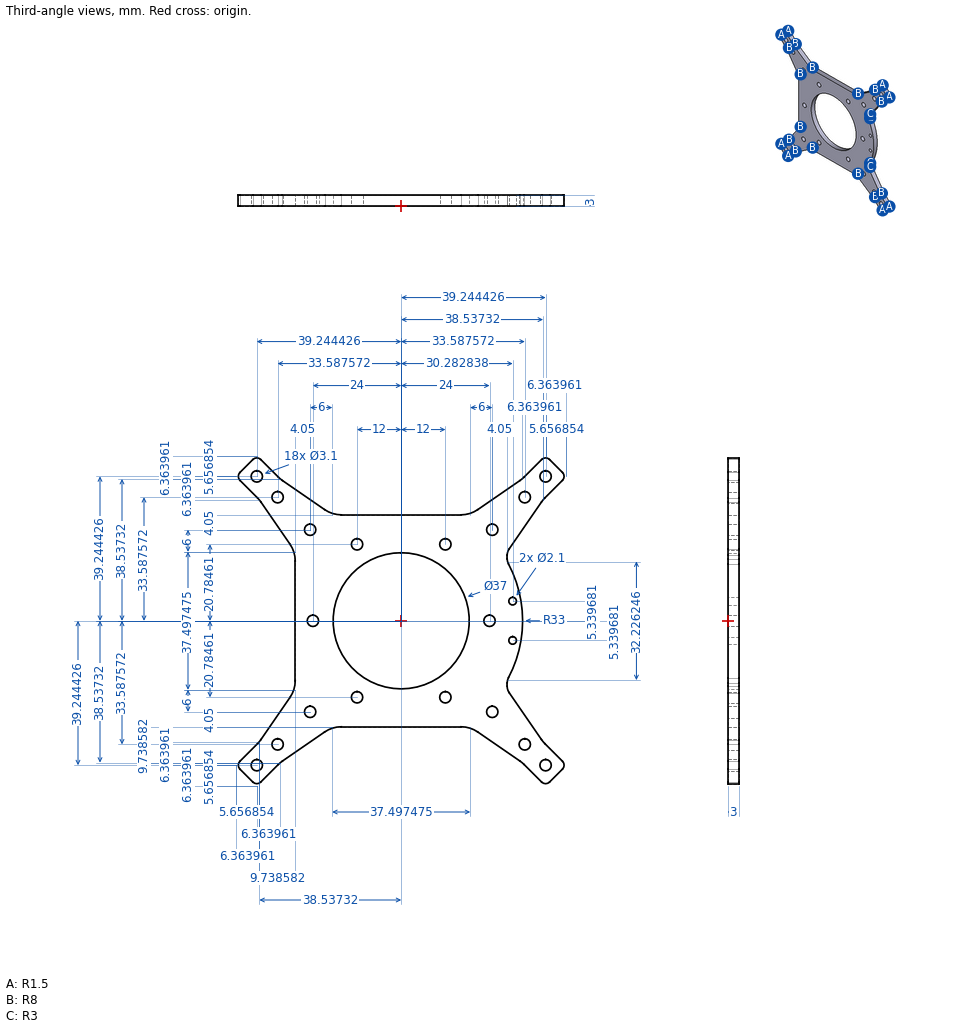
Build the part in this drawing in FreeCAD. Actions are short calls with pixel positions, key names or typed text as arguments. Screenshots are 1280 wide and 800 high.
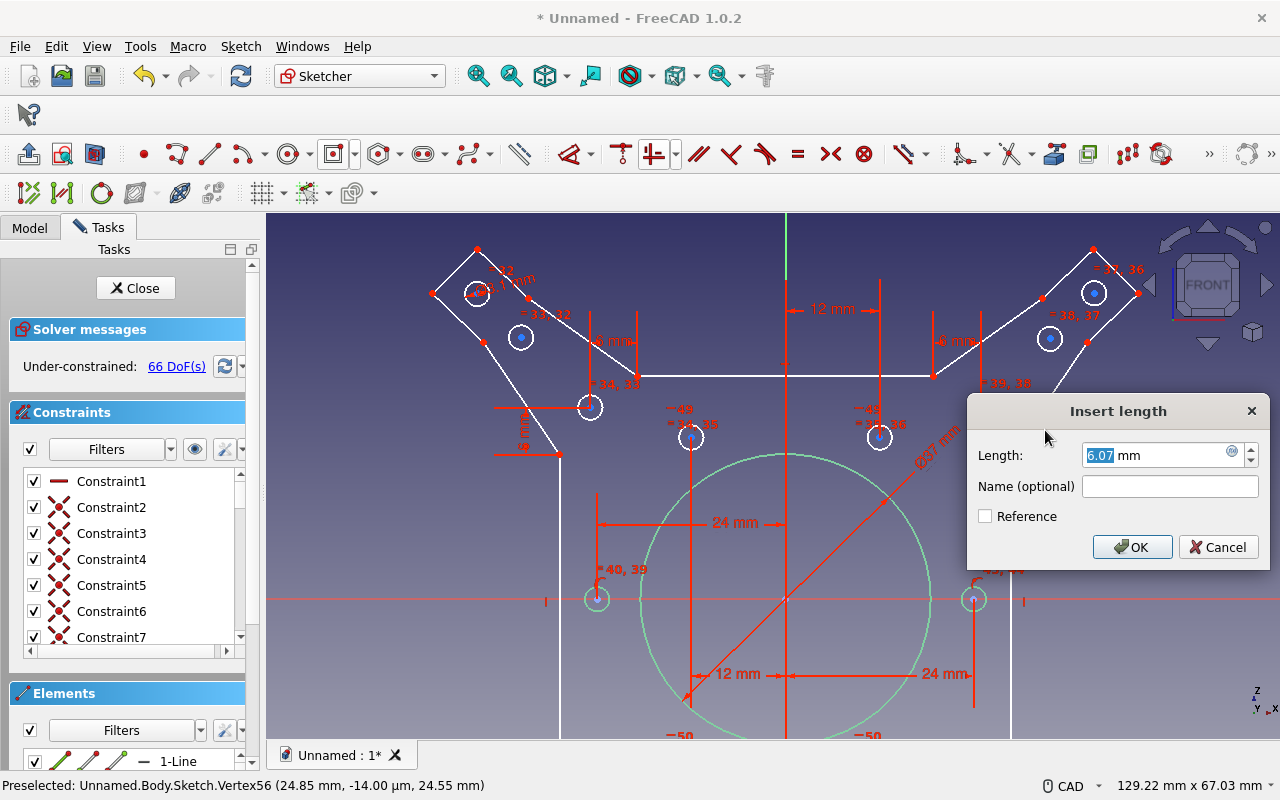
text(6)
key(Return)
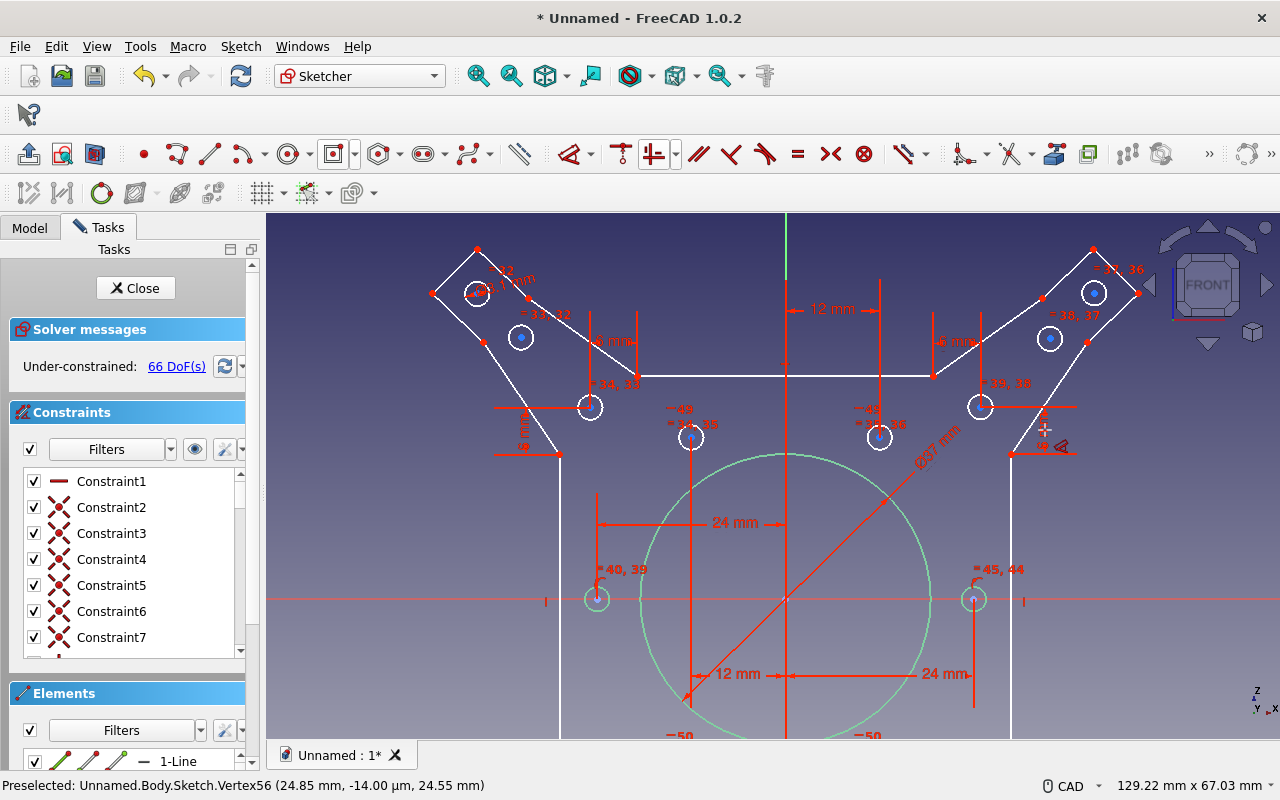
scroll(638, 375, down, 4)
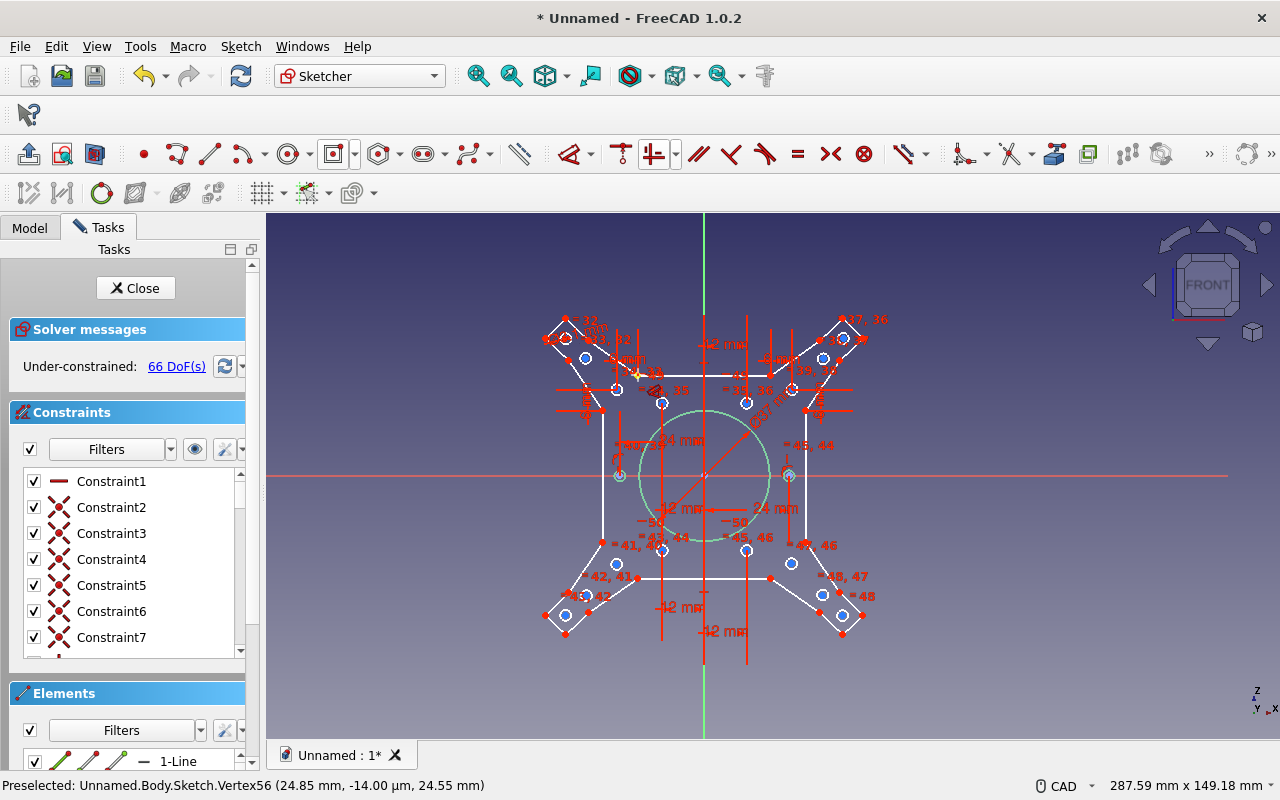
scroll(638, 579, up, 4)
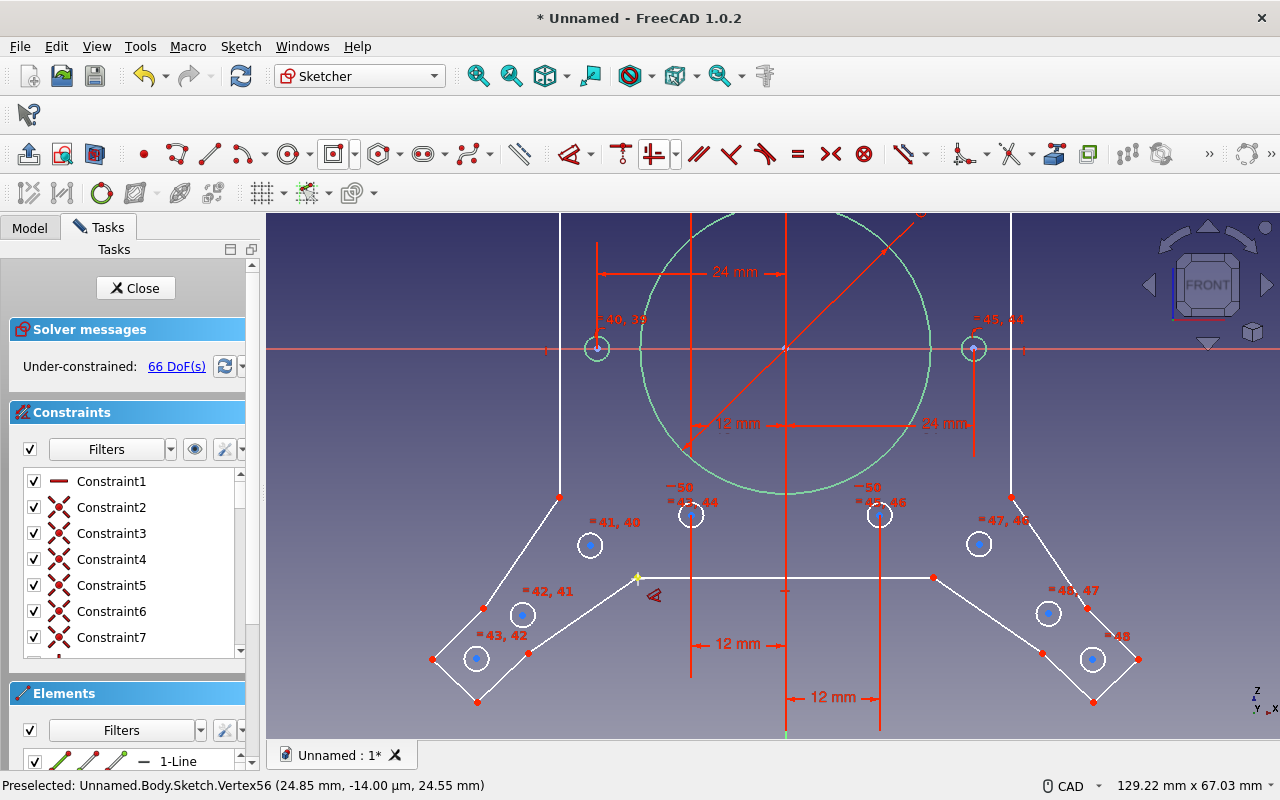
click(637, 578)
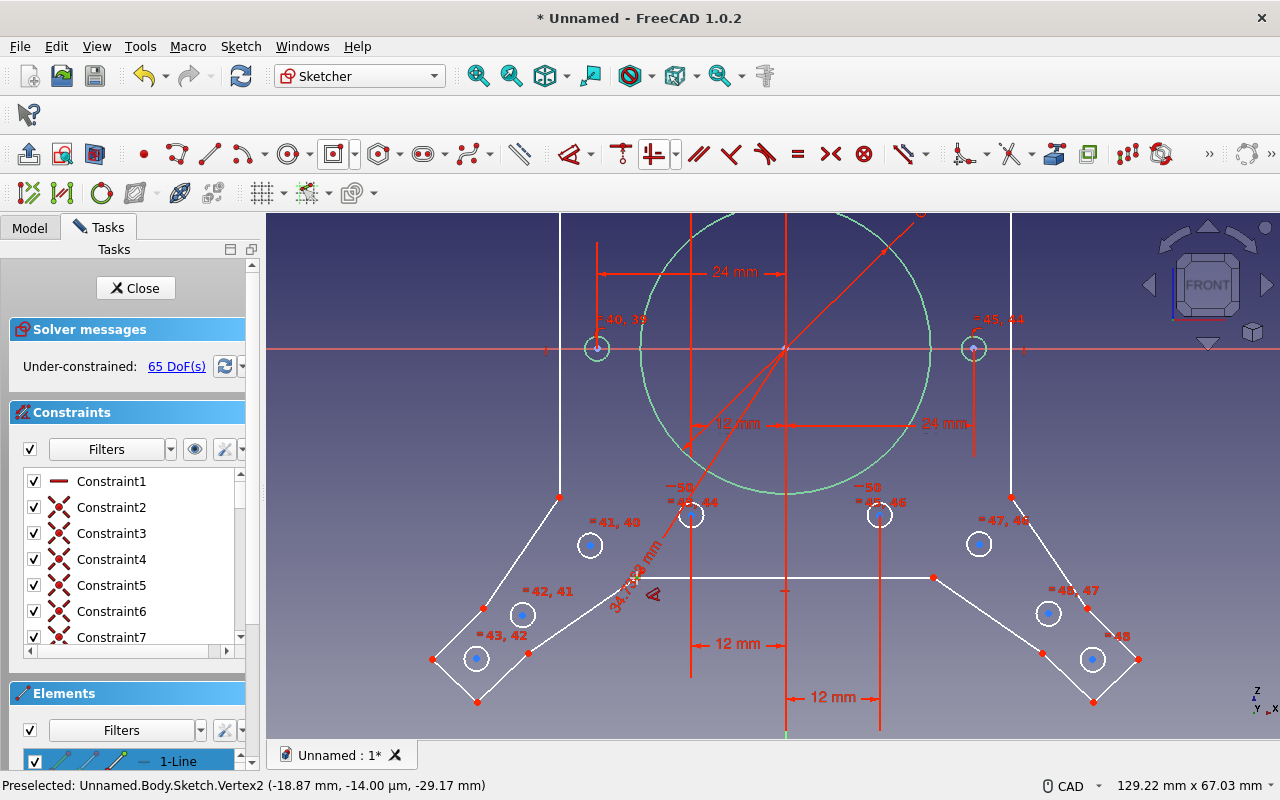
click(590, 546)
click(614, 612)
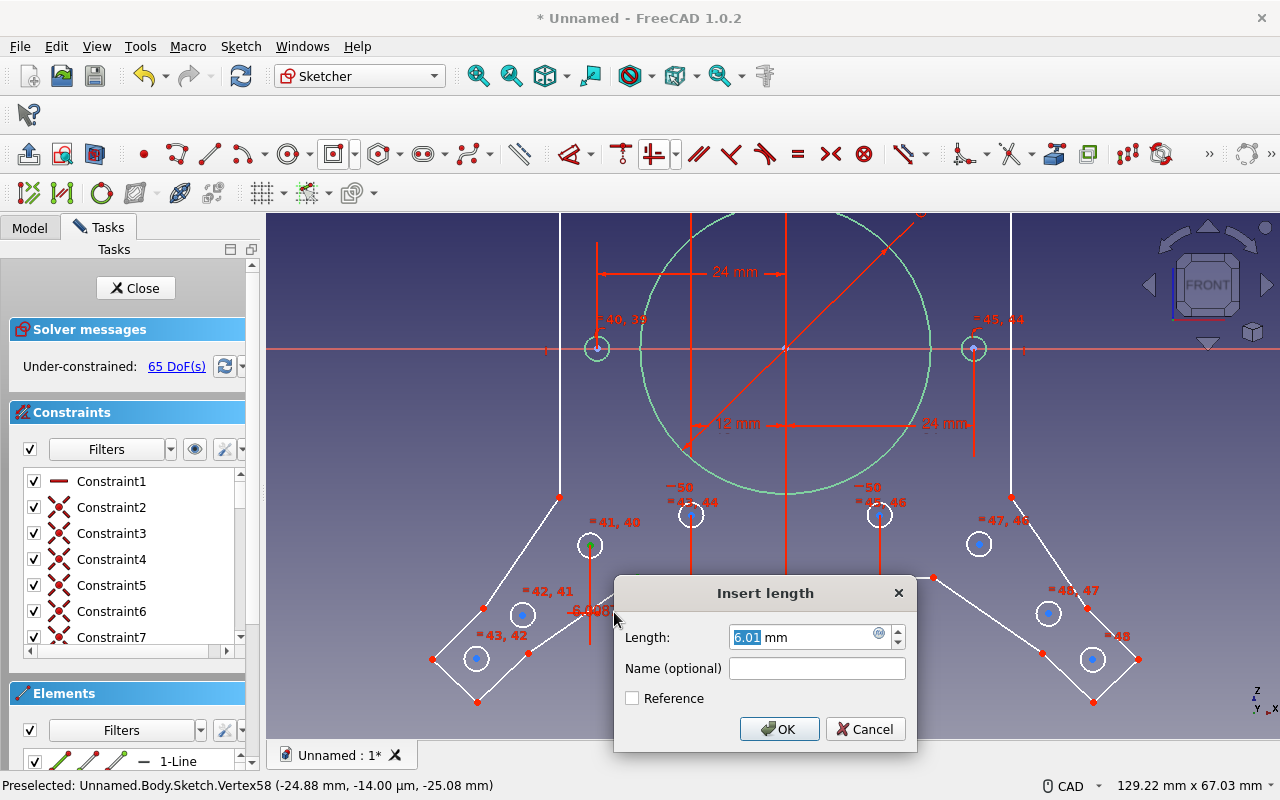
text(6)
key(Return)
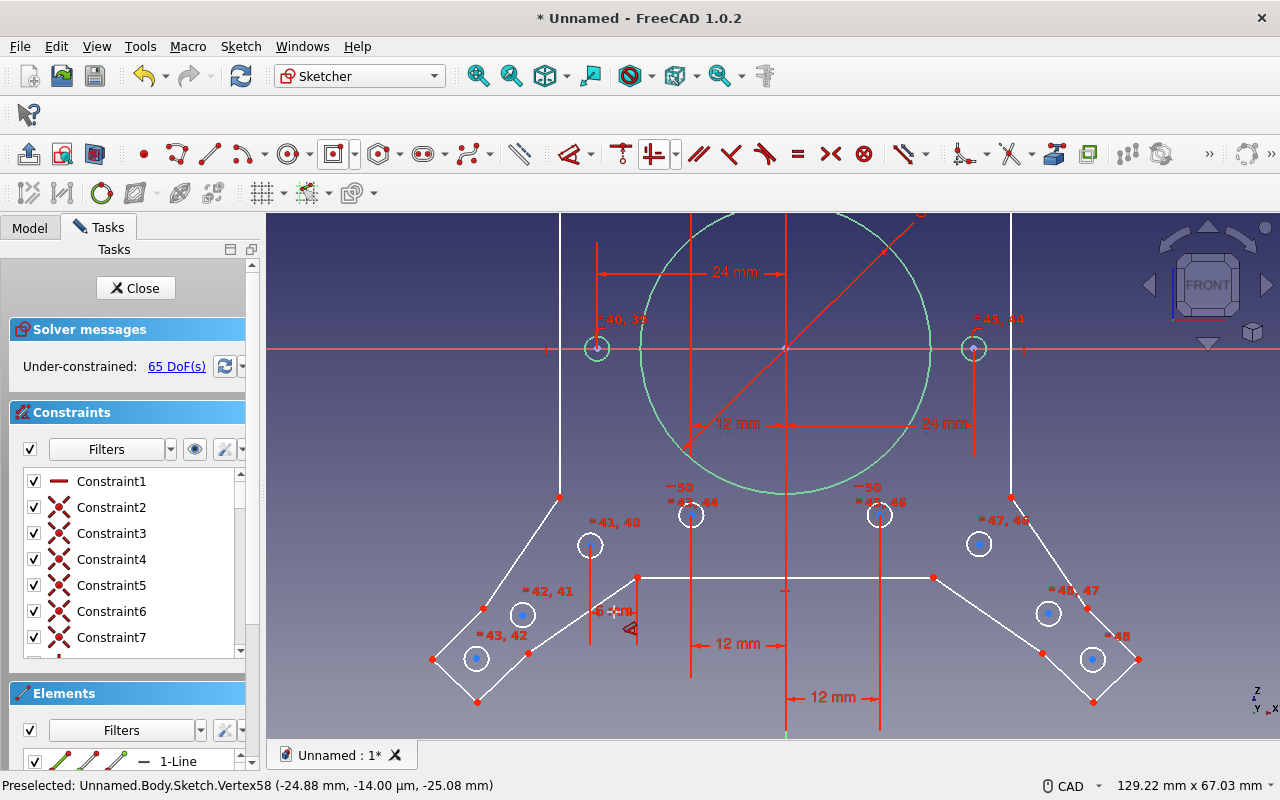
click(560, 498)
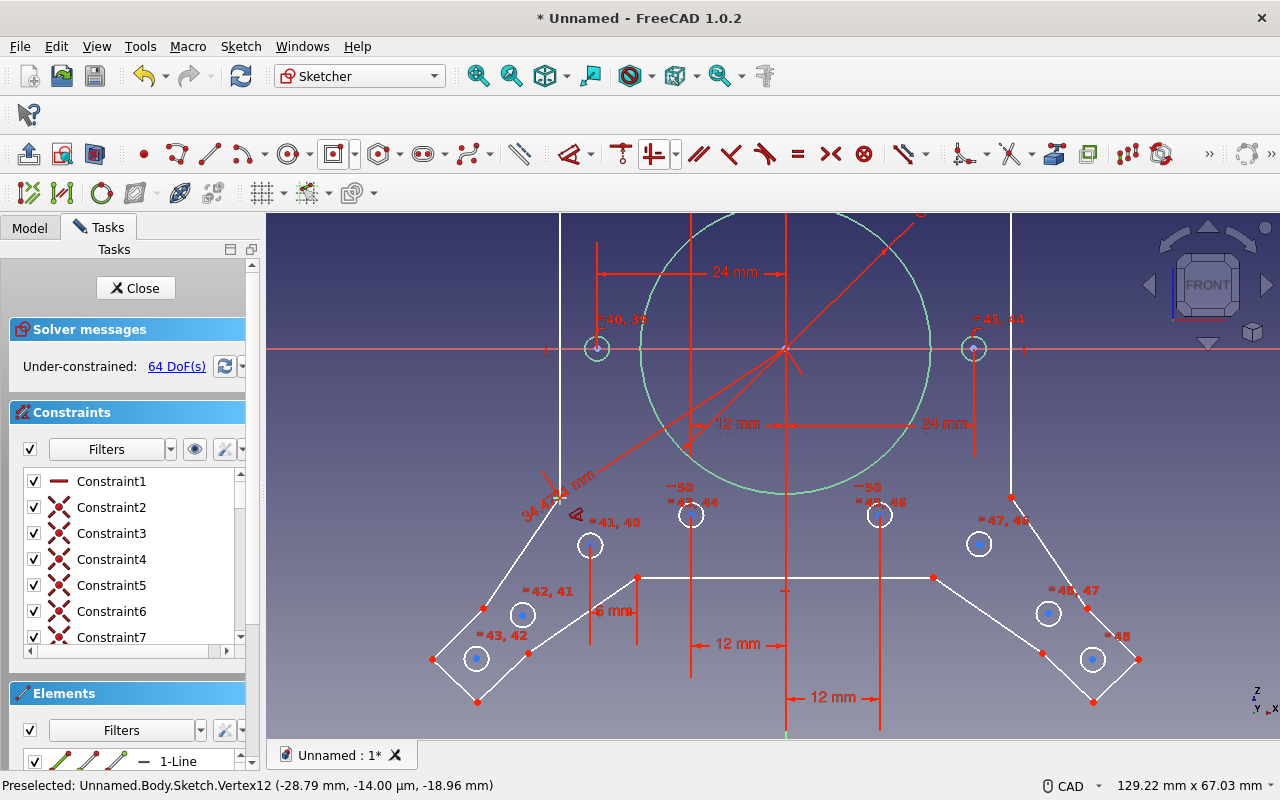
click(590, 546)
click(526, 522)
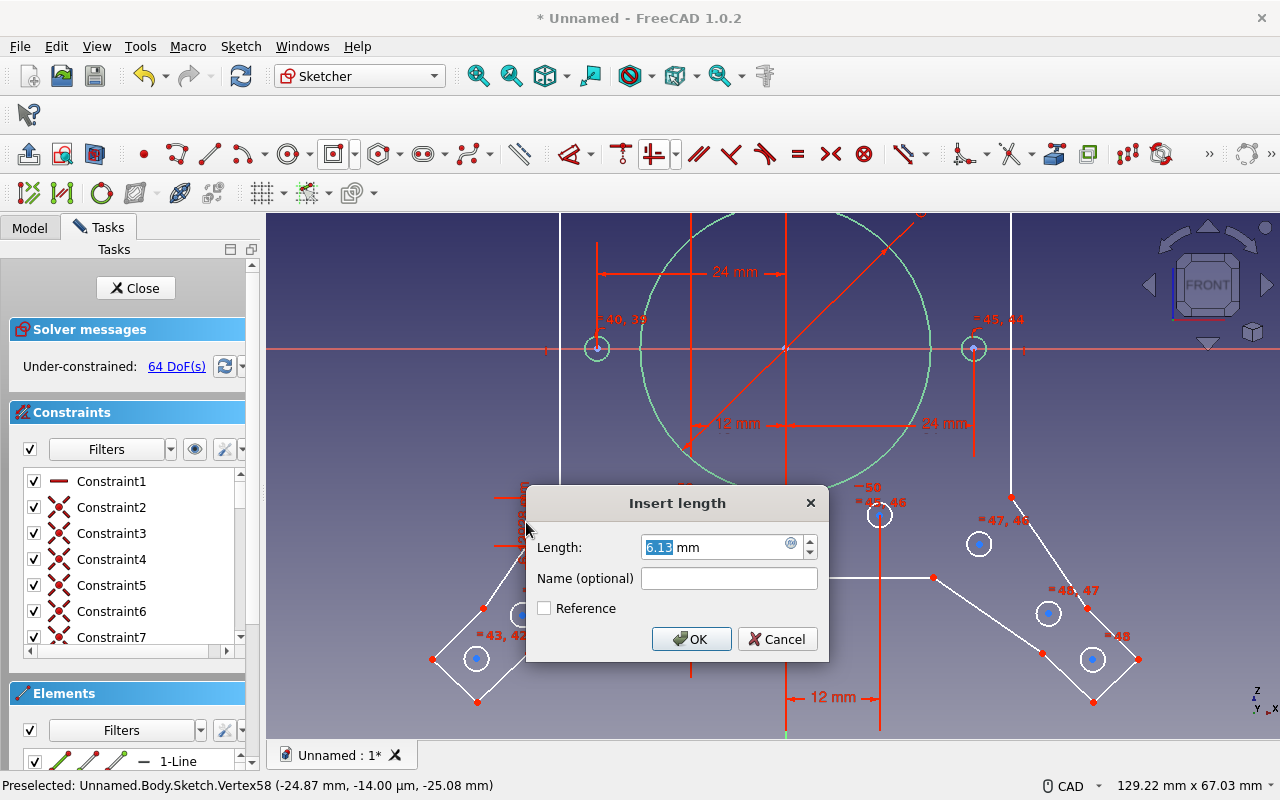
text(6)
key(Return)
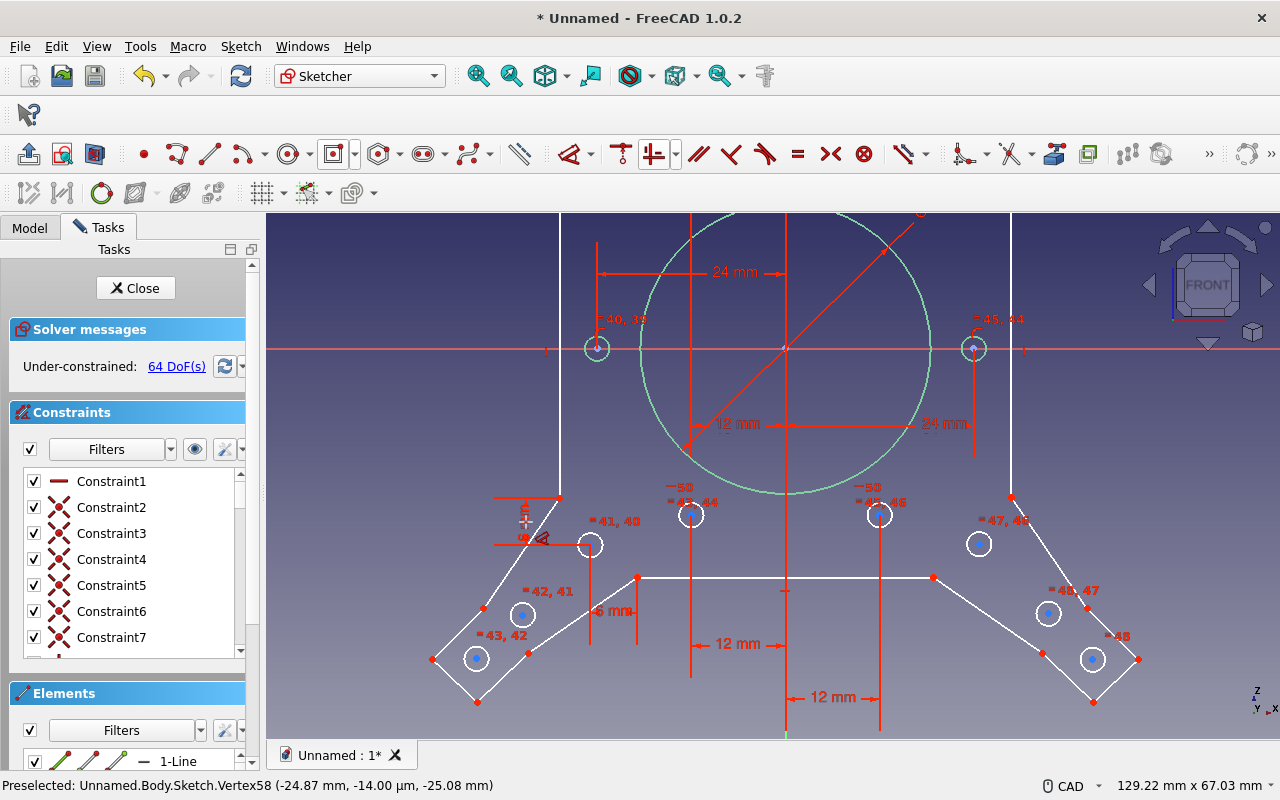
click(933, 578)